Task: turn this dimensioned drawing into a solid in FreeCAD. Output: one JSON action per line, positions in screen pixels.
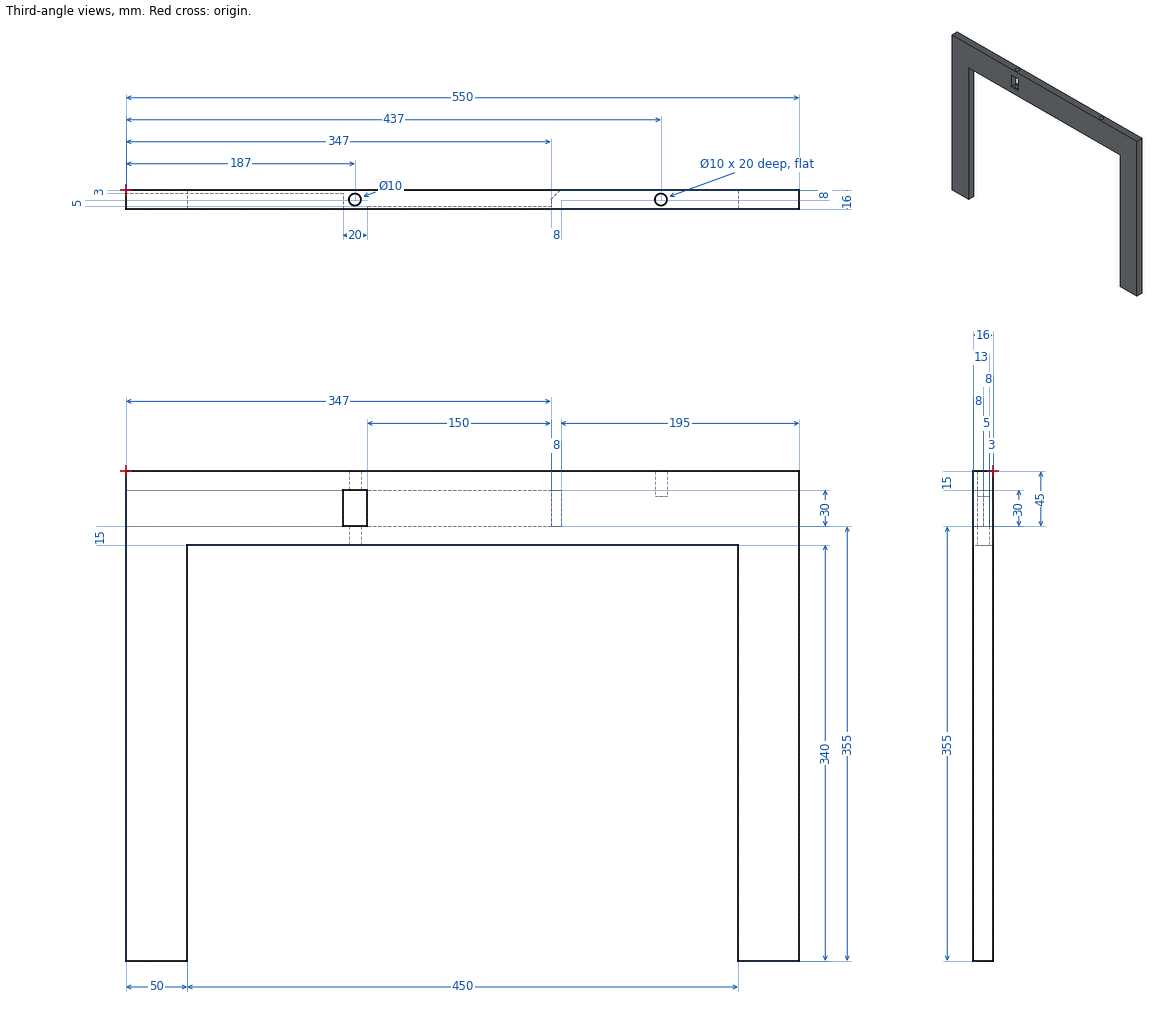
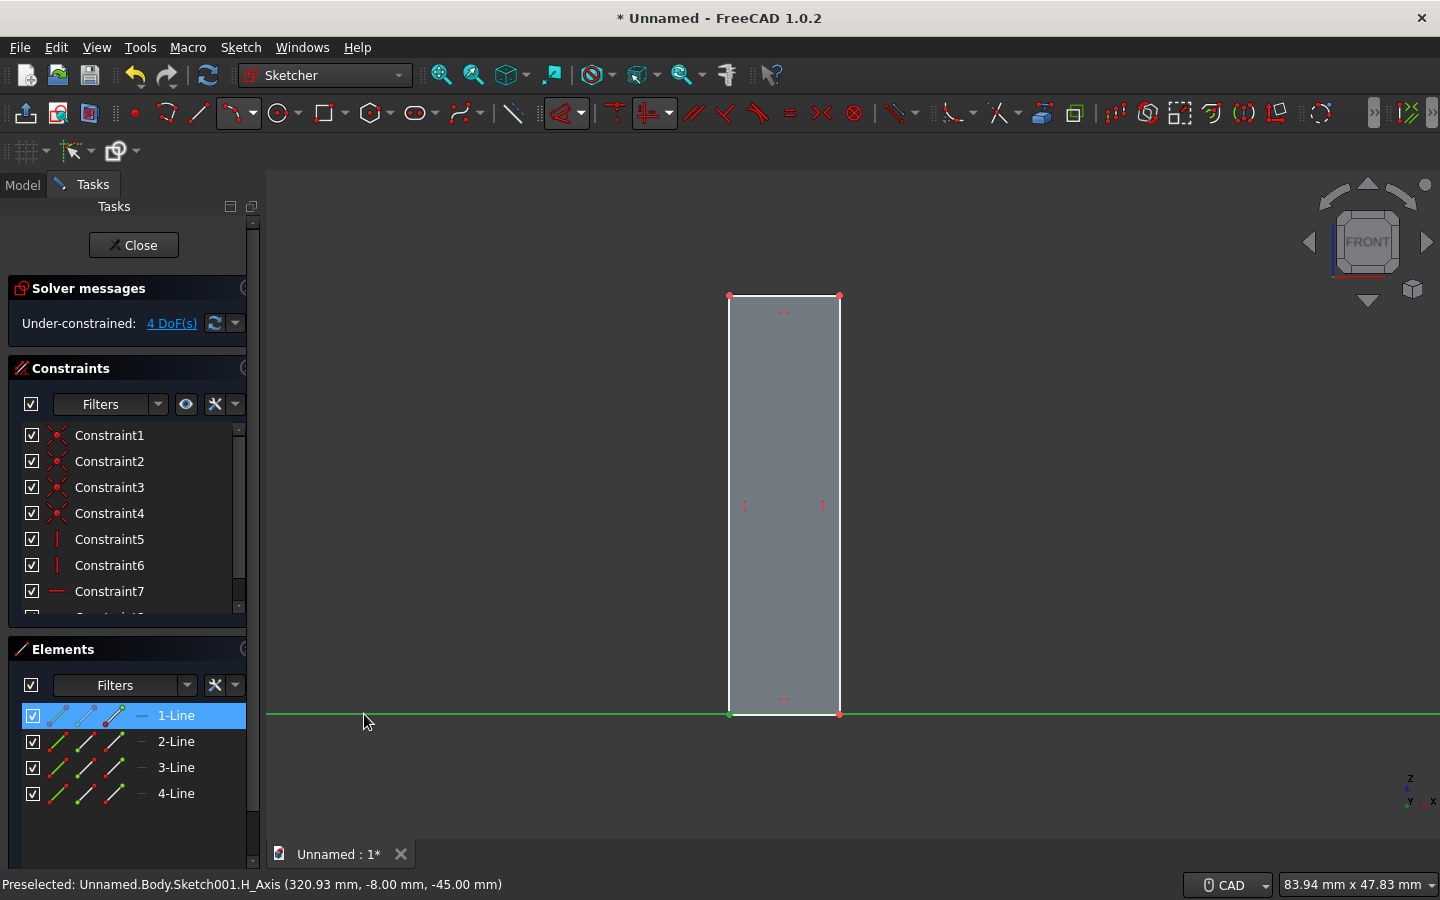
{"action": "left_click", "coordinate": [616, 114]}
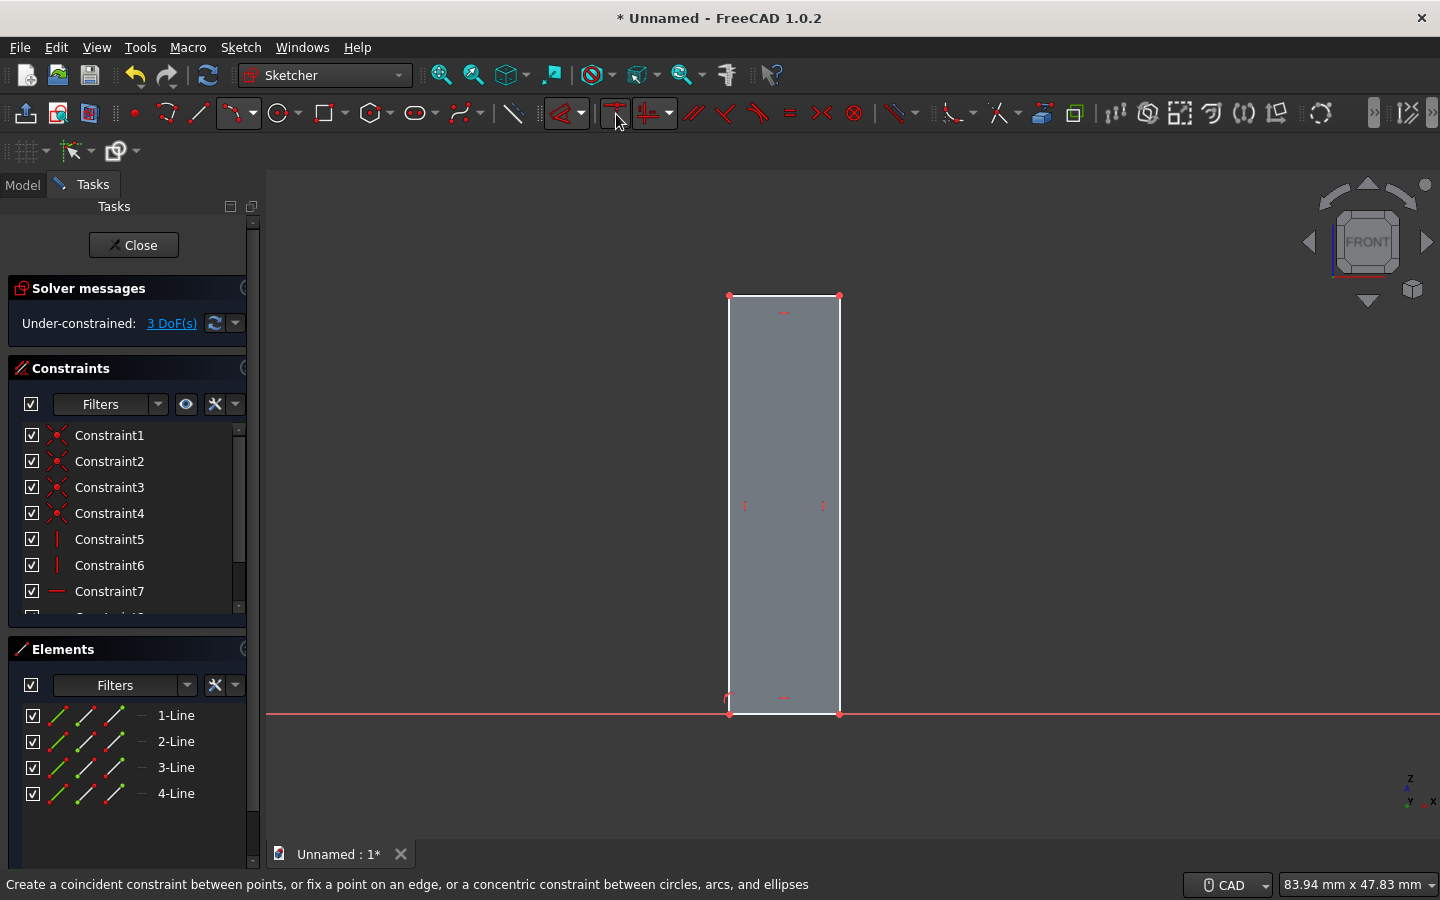
{"action": "left_click", "coordinate": [762, 714]}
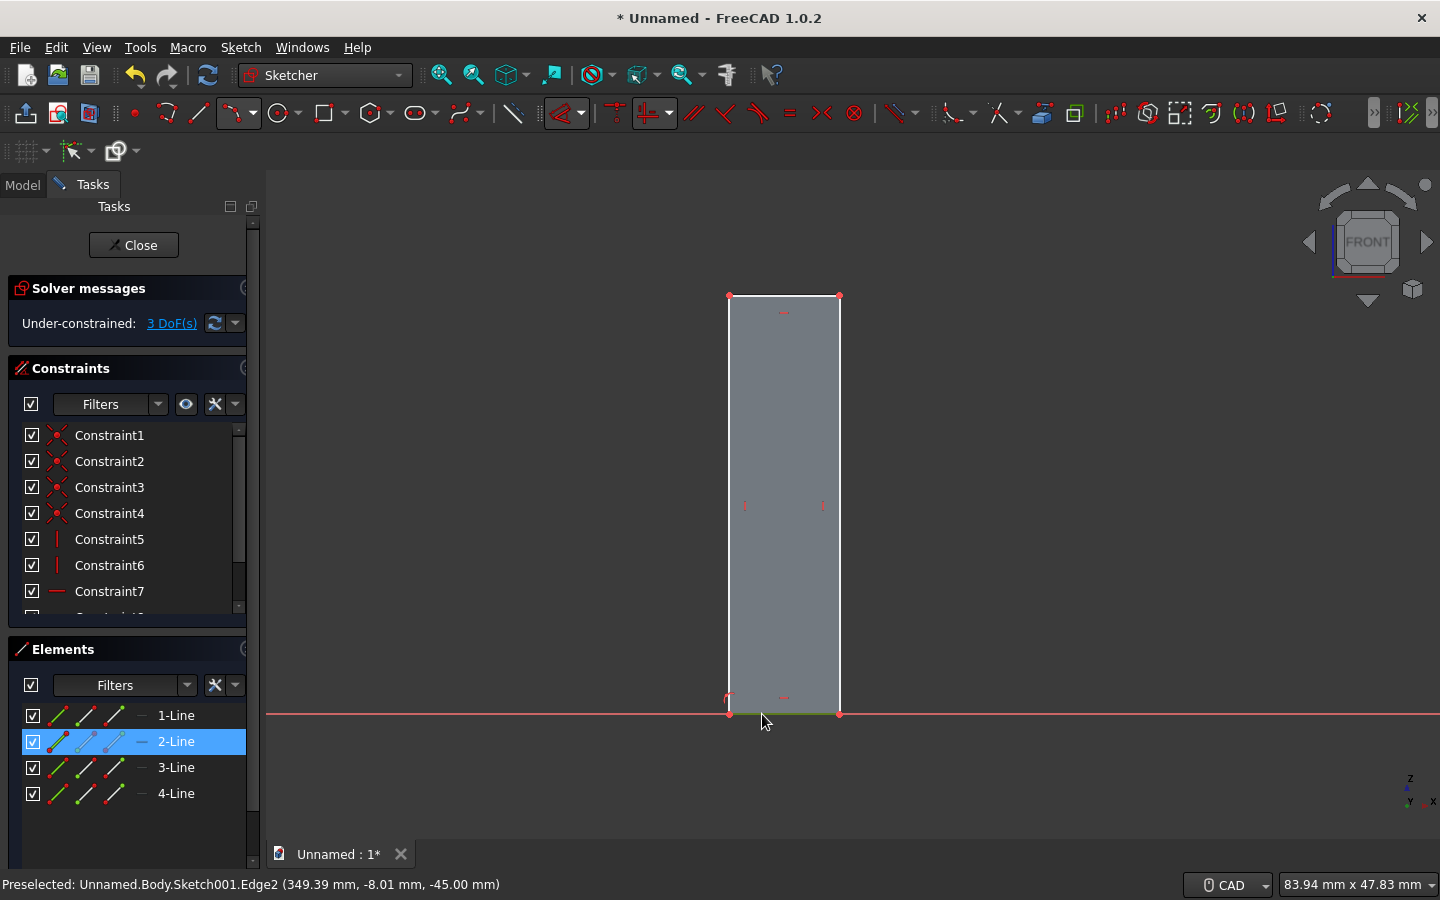
{"action": "left_click", "coordinate": [584, 114]}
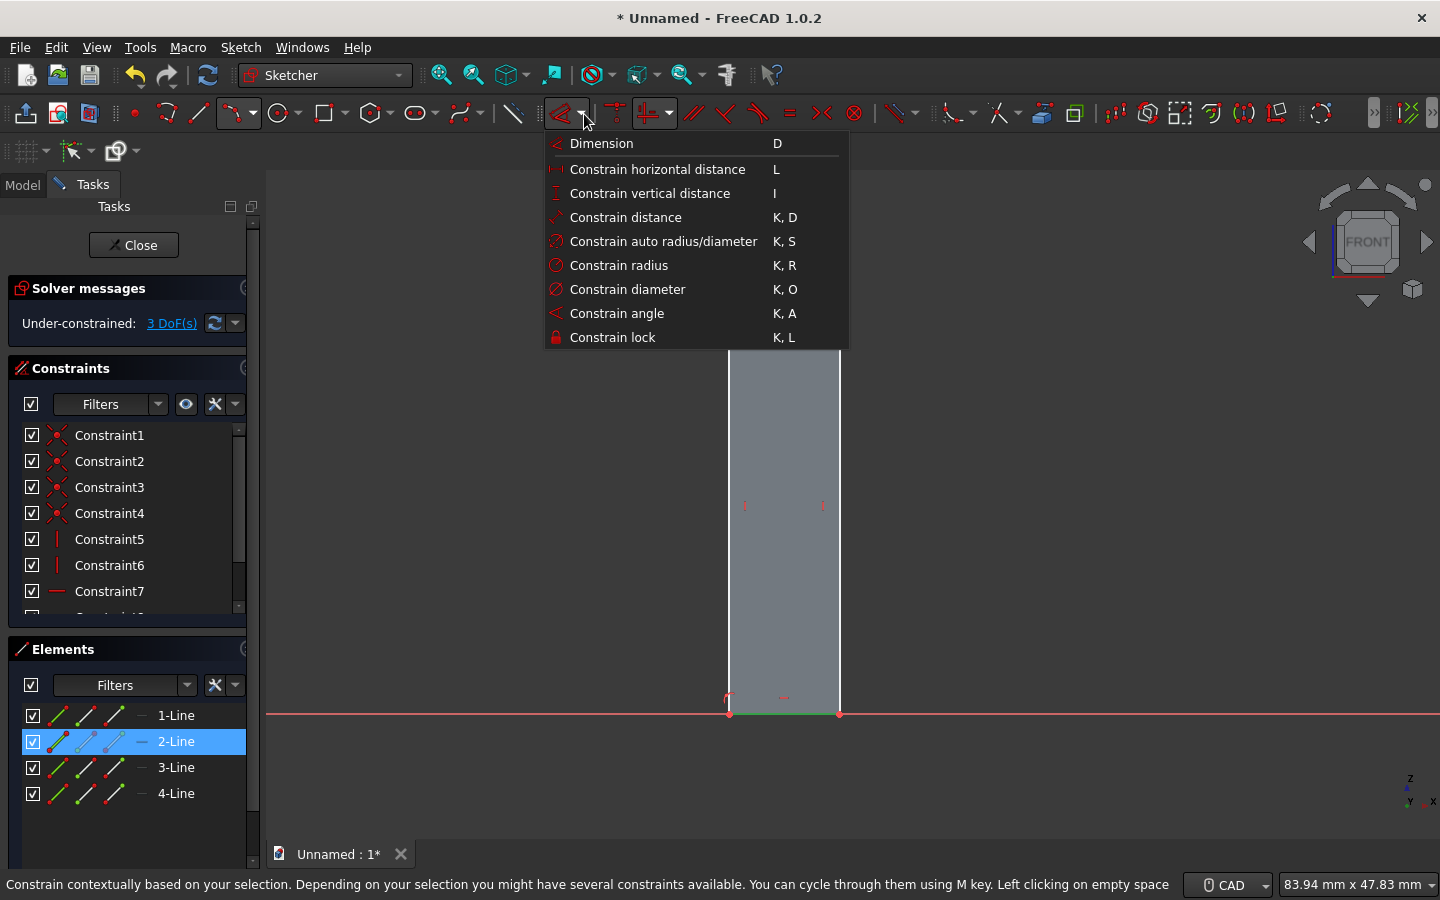
{"action": "left_click", "coordinate": [697, 169]}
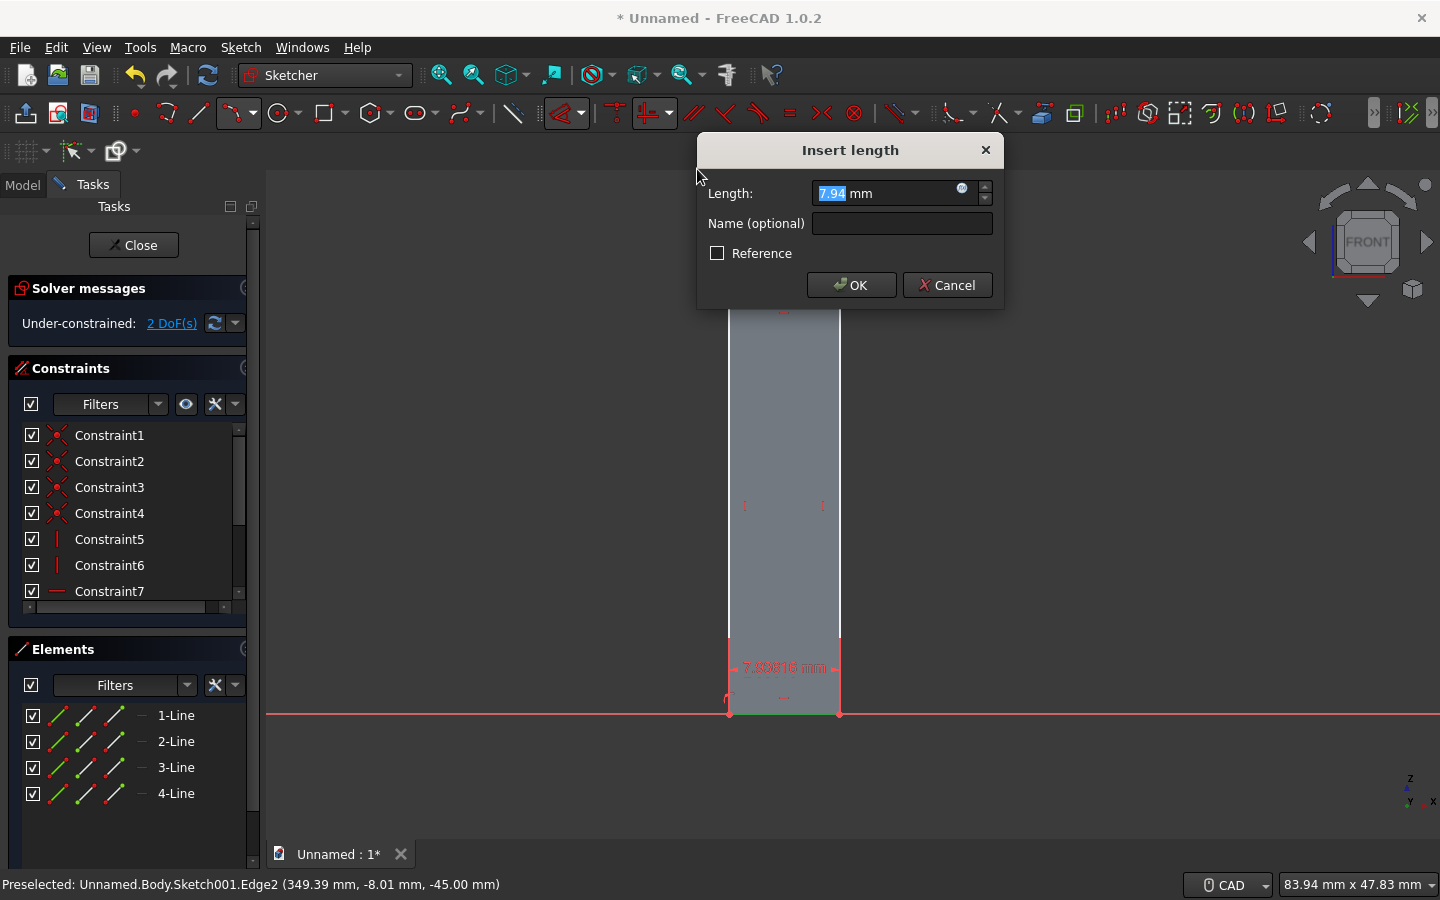
{"action": "type", "text": "8"}
{"action": "key", "text": "Return"}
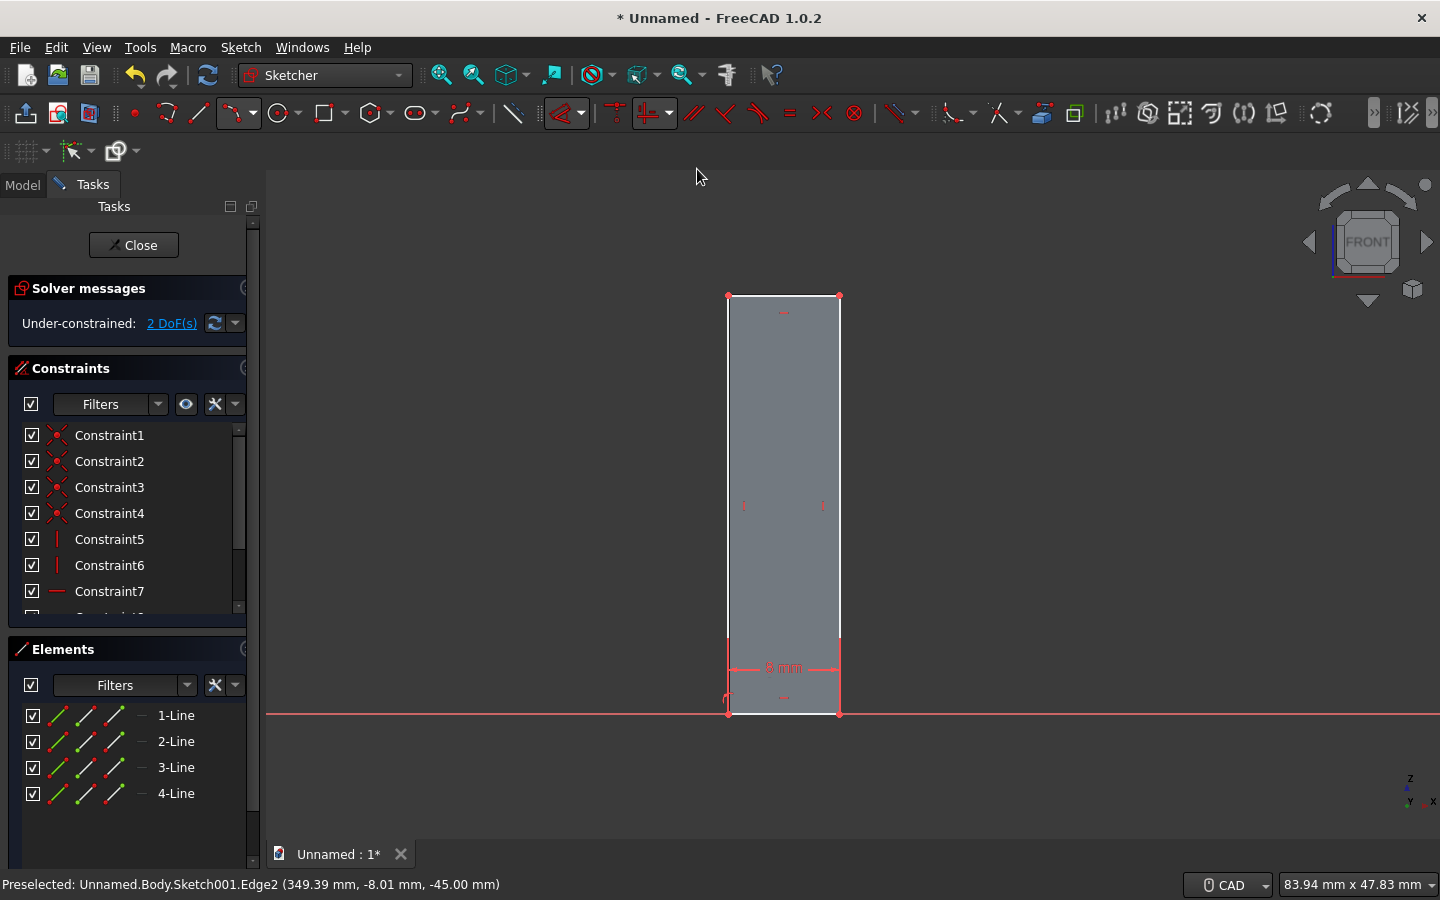
{"action": "left_click", "coordinate": [728, 421]}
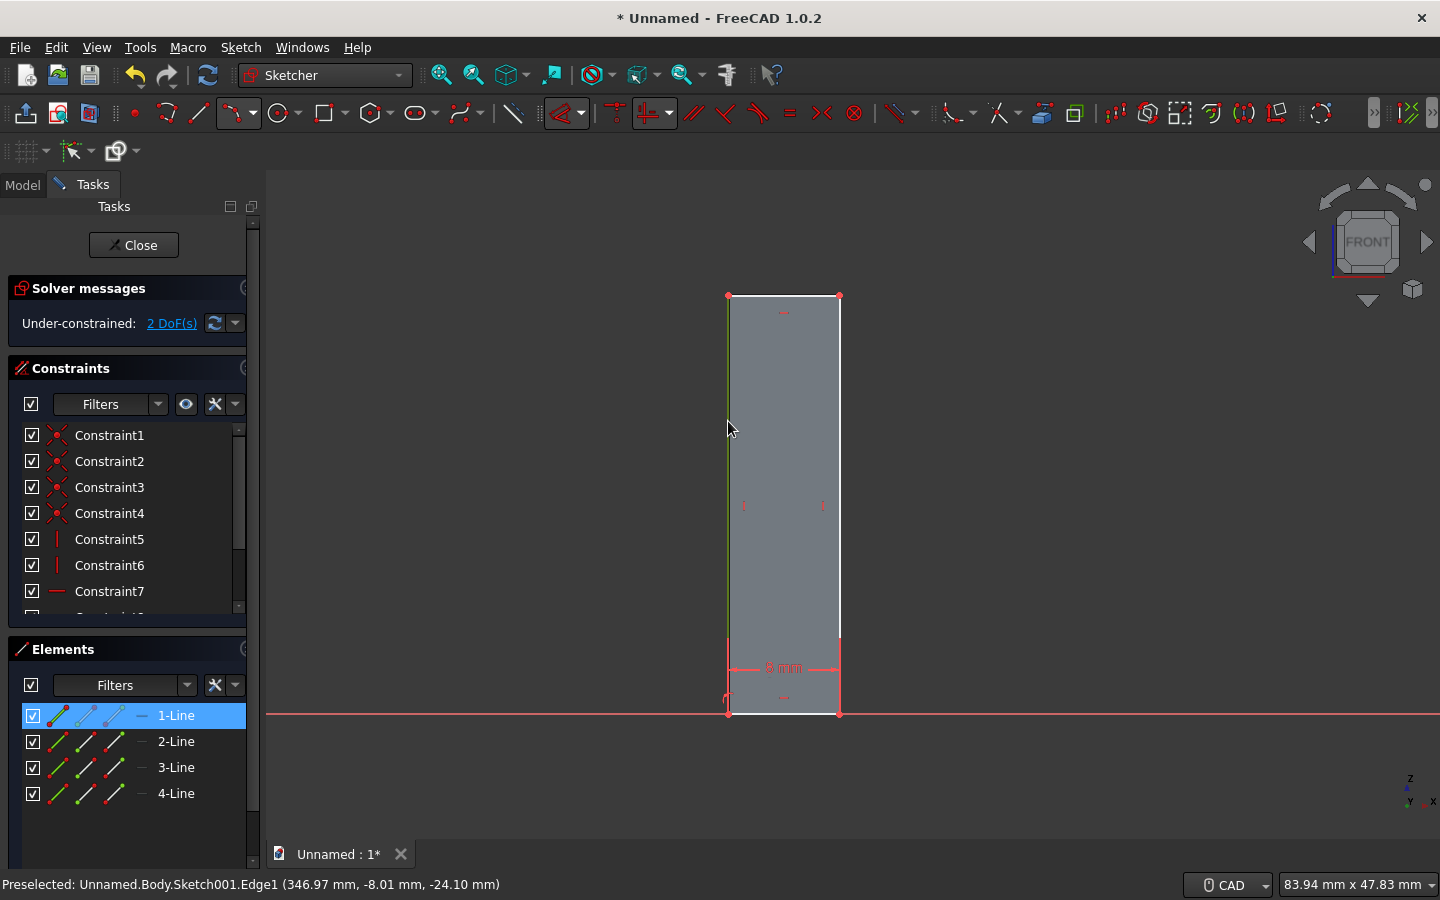
{"action": "key", "text": "i"}